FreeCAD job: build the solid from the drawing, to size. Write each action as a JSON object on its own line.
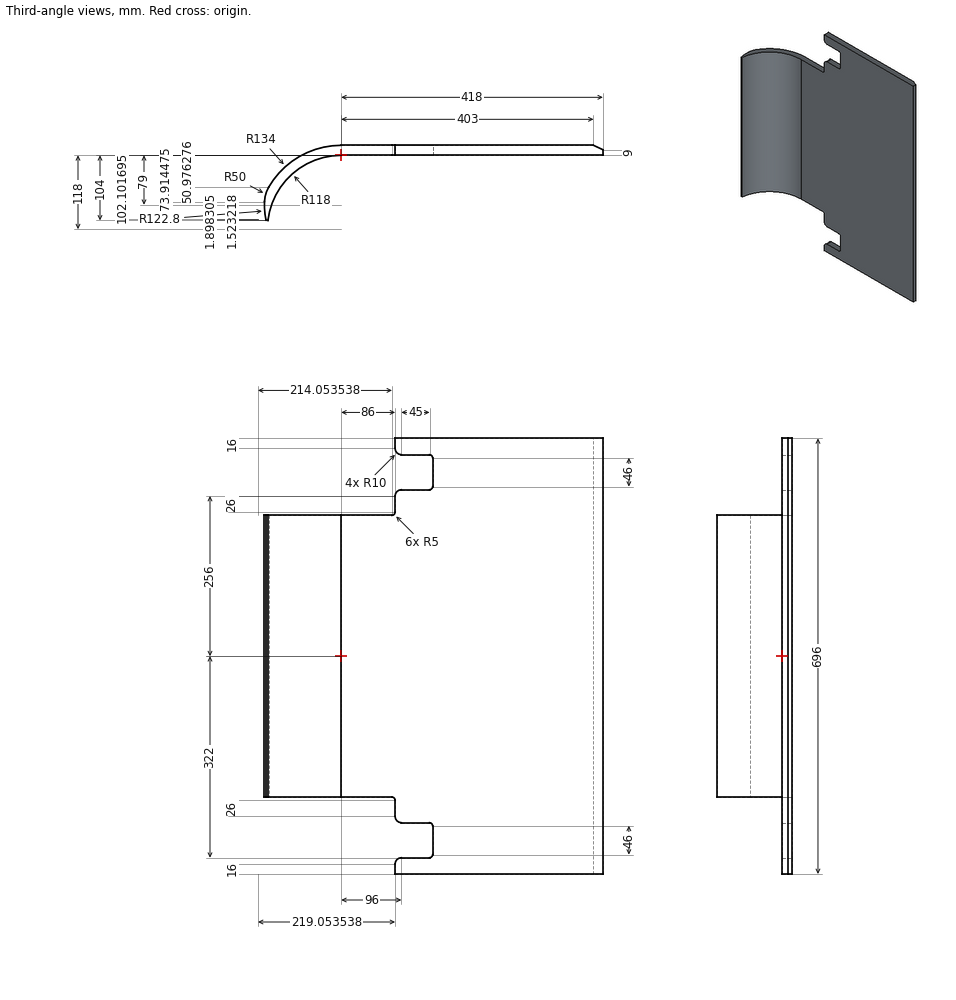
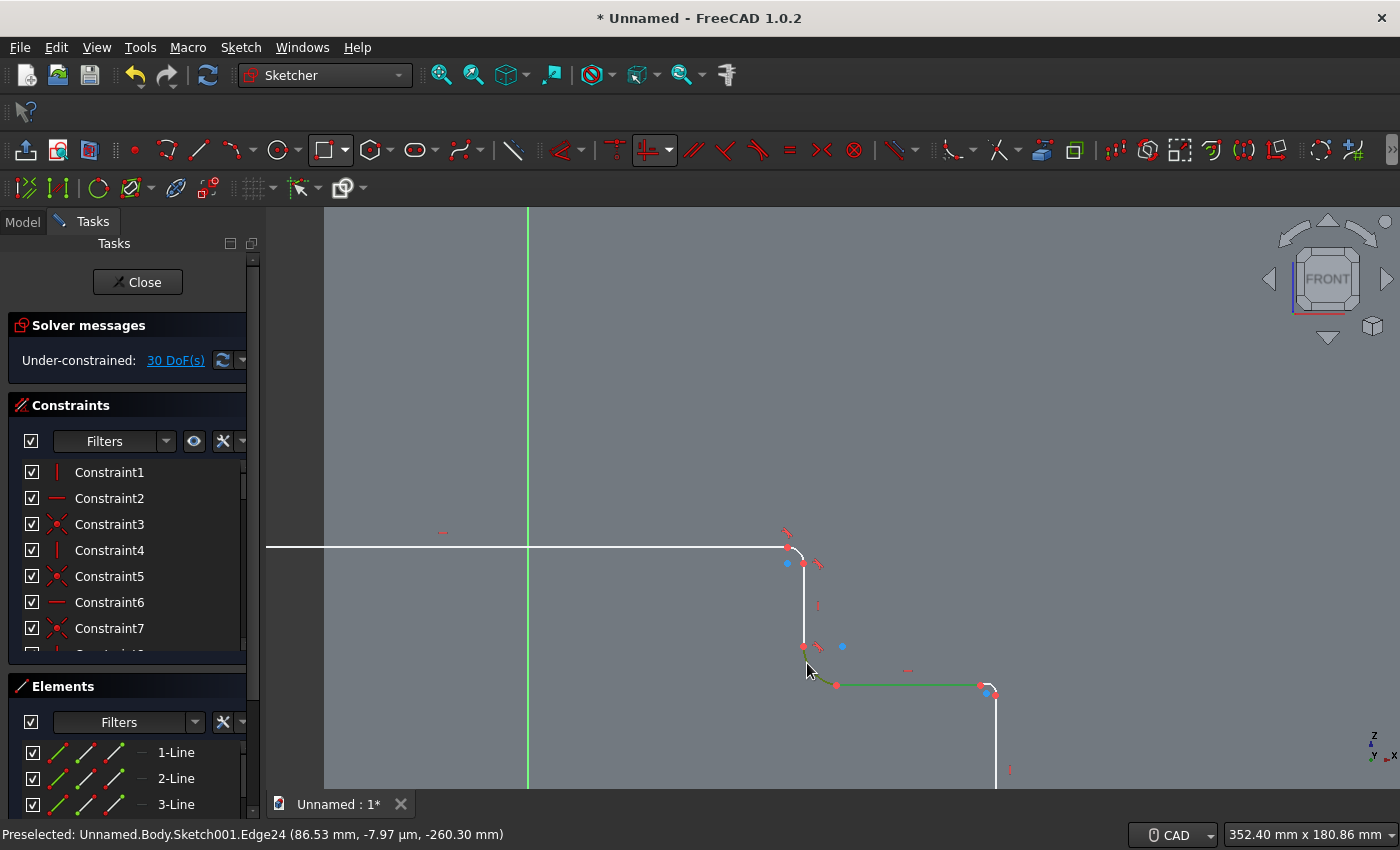
{"action": "left_click", "coordinate": [758, 150]}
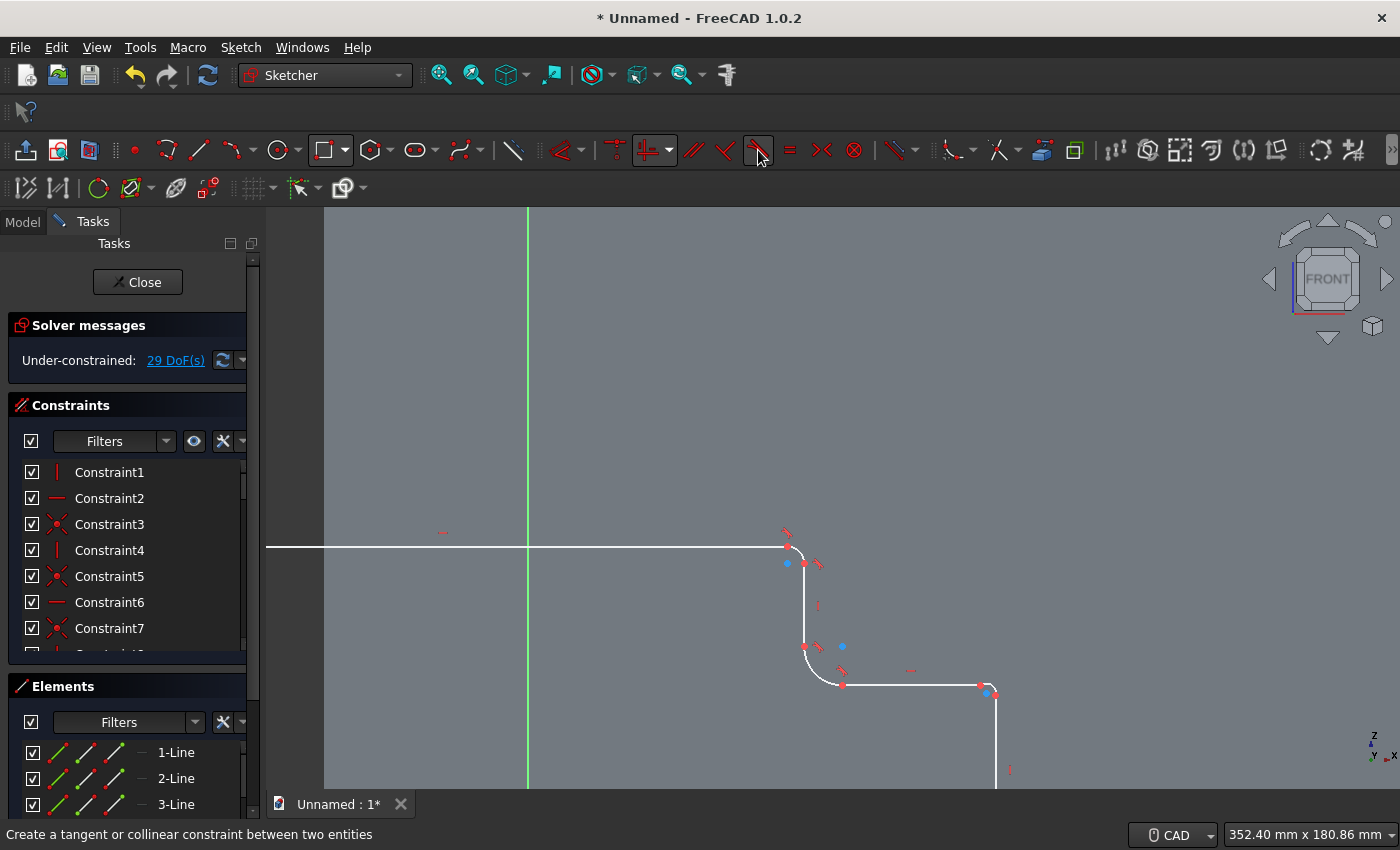
{"action": "scroll", "coordinate": [807, 632], "scroll_direction": "down", "scroll_amount": 9}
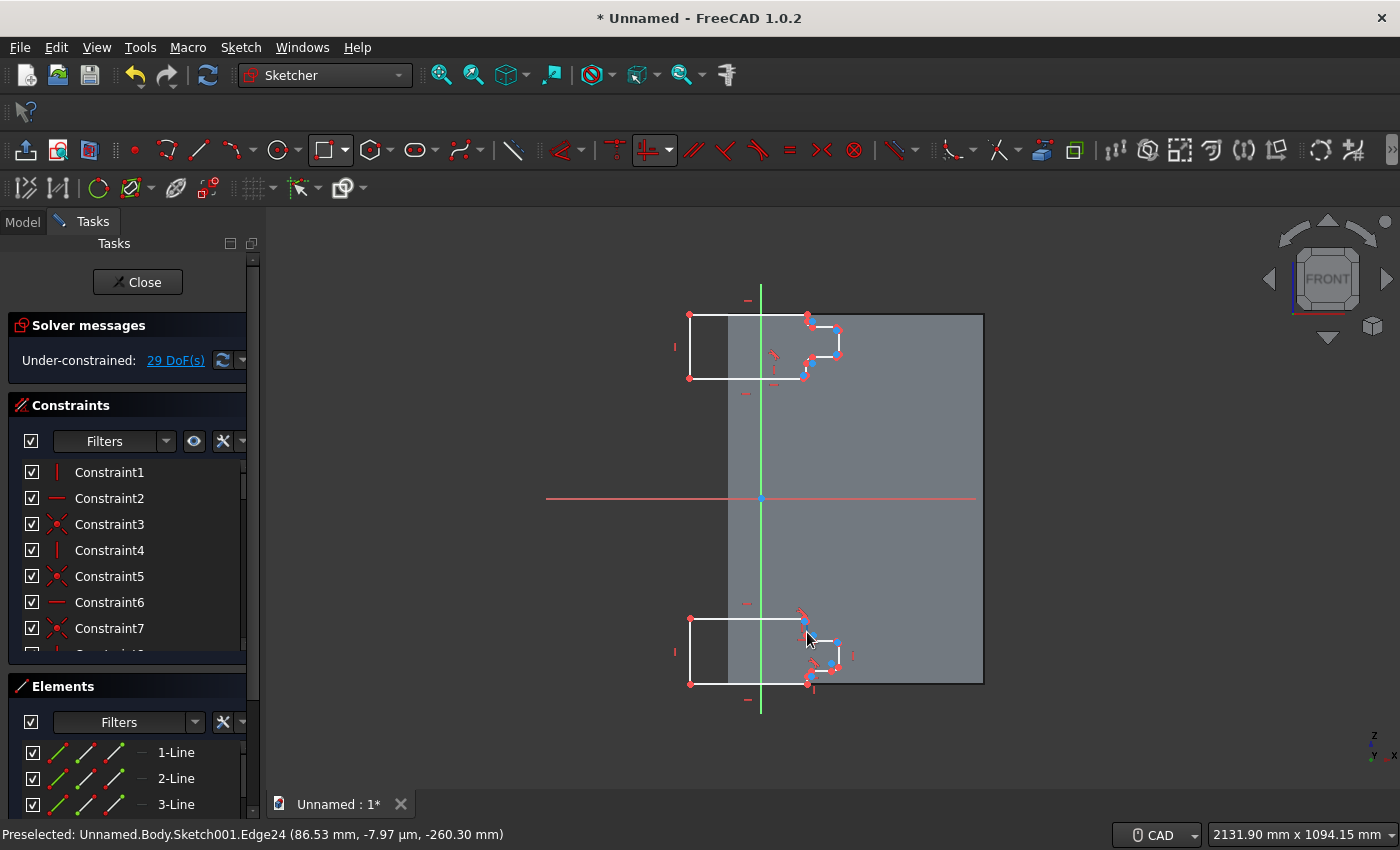
{"action": "scroll", "coordinate": [820, 641], "scroll_direction": "up", "scroll_amount": 4}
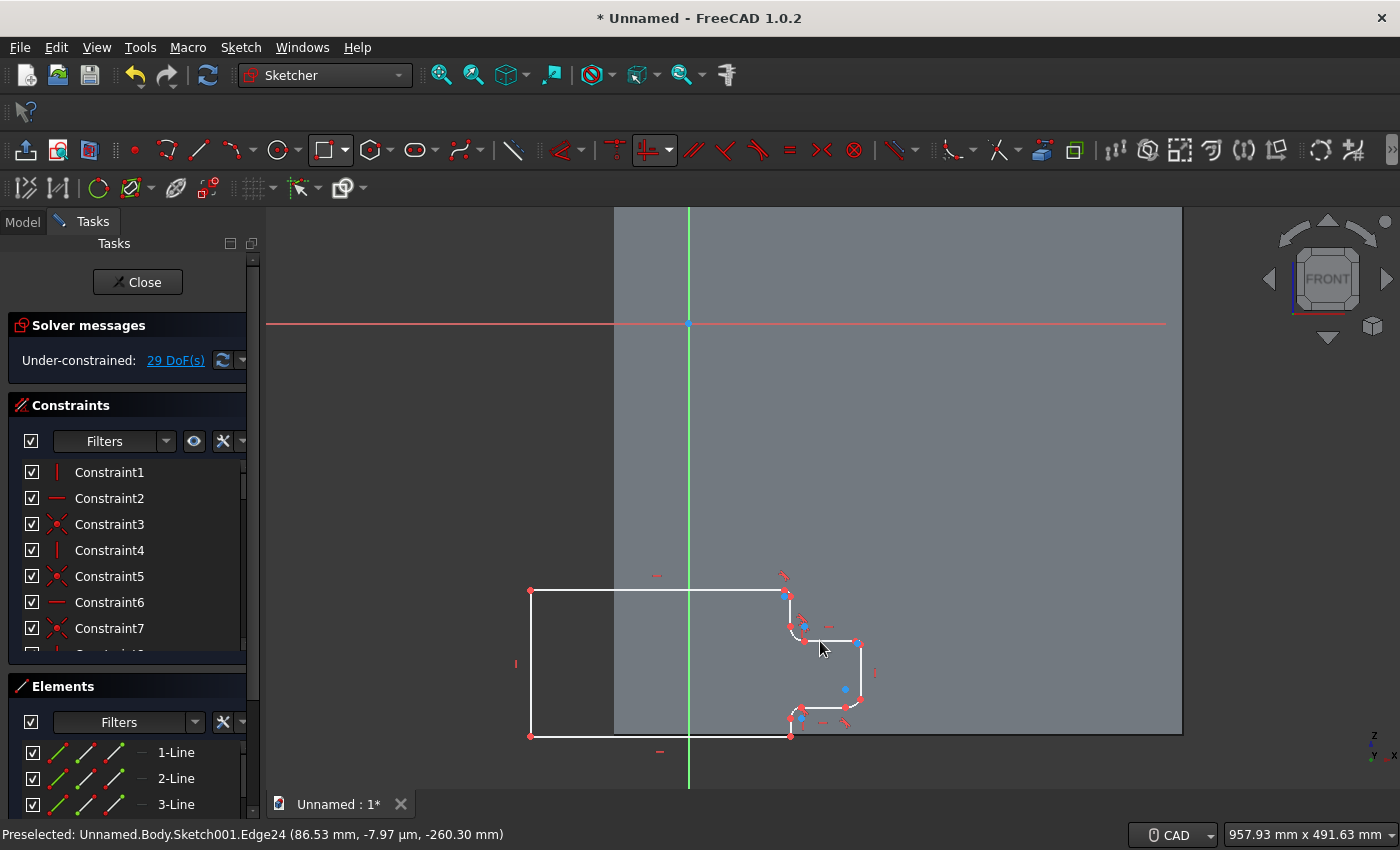
{"action": "left_click", "coordinate": [820, 641]}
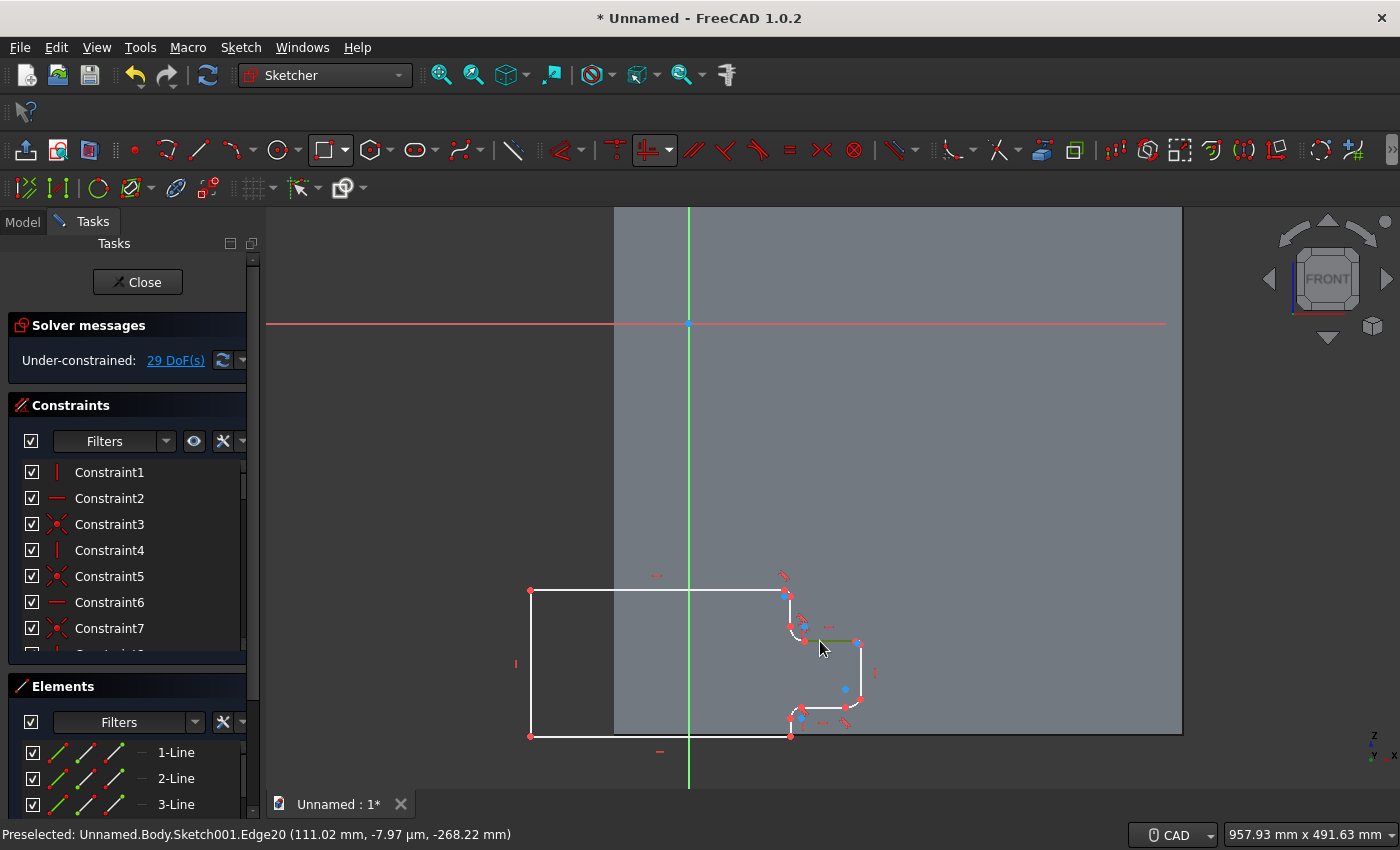
{"action": "scroll", "coordinate": [859, 641], "scroll_direction": "up", "scroll_amount": 7}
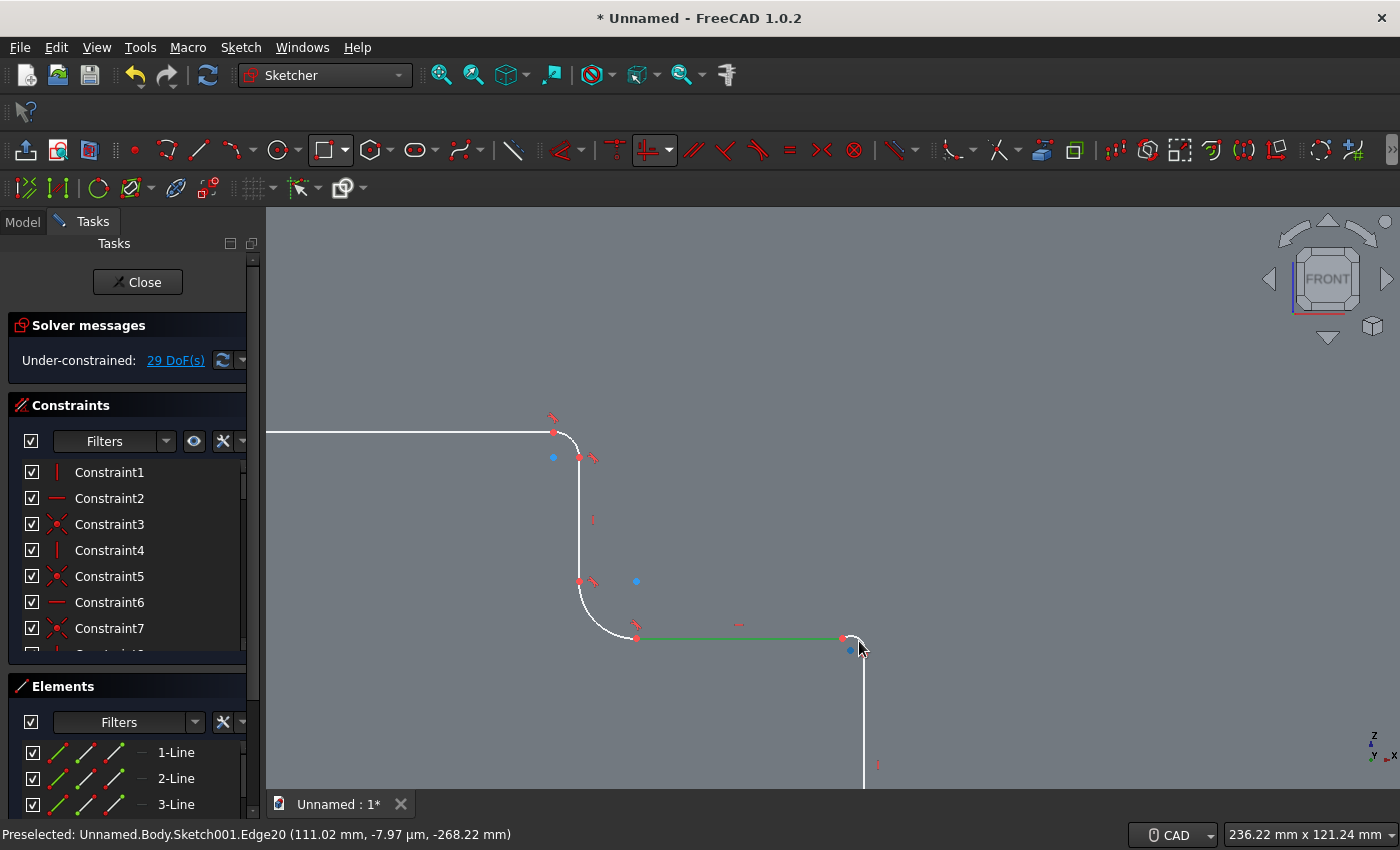
{"action": "left_click", "coordinate": [859, 639]}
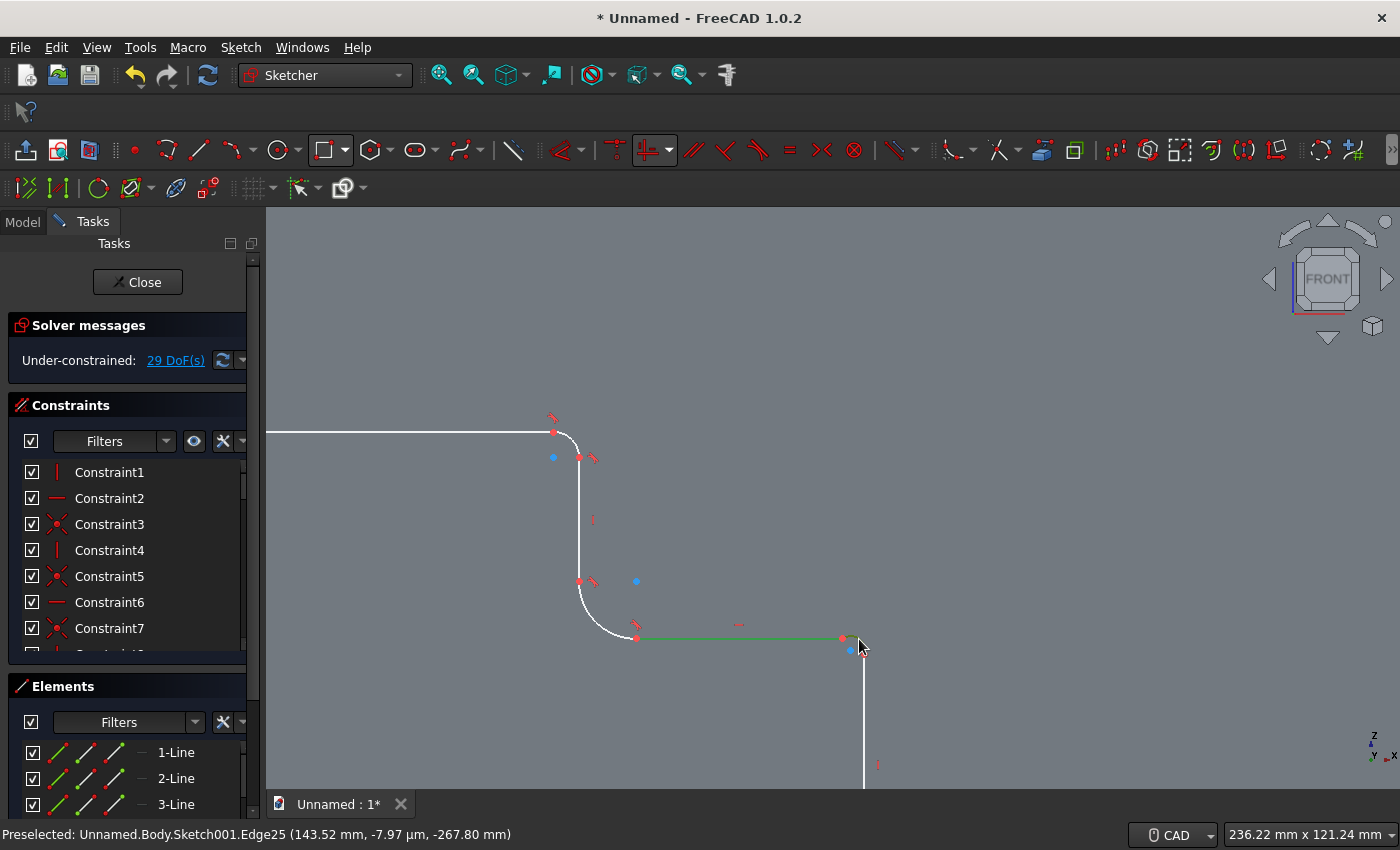
{"action": "left_click", "coordinate": [758, 150]}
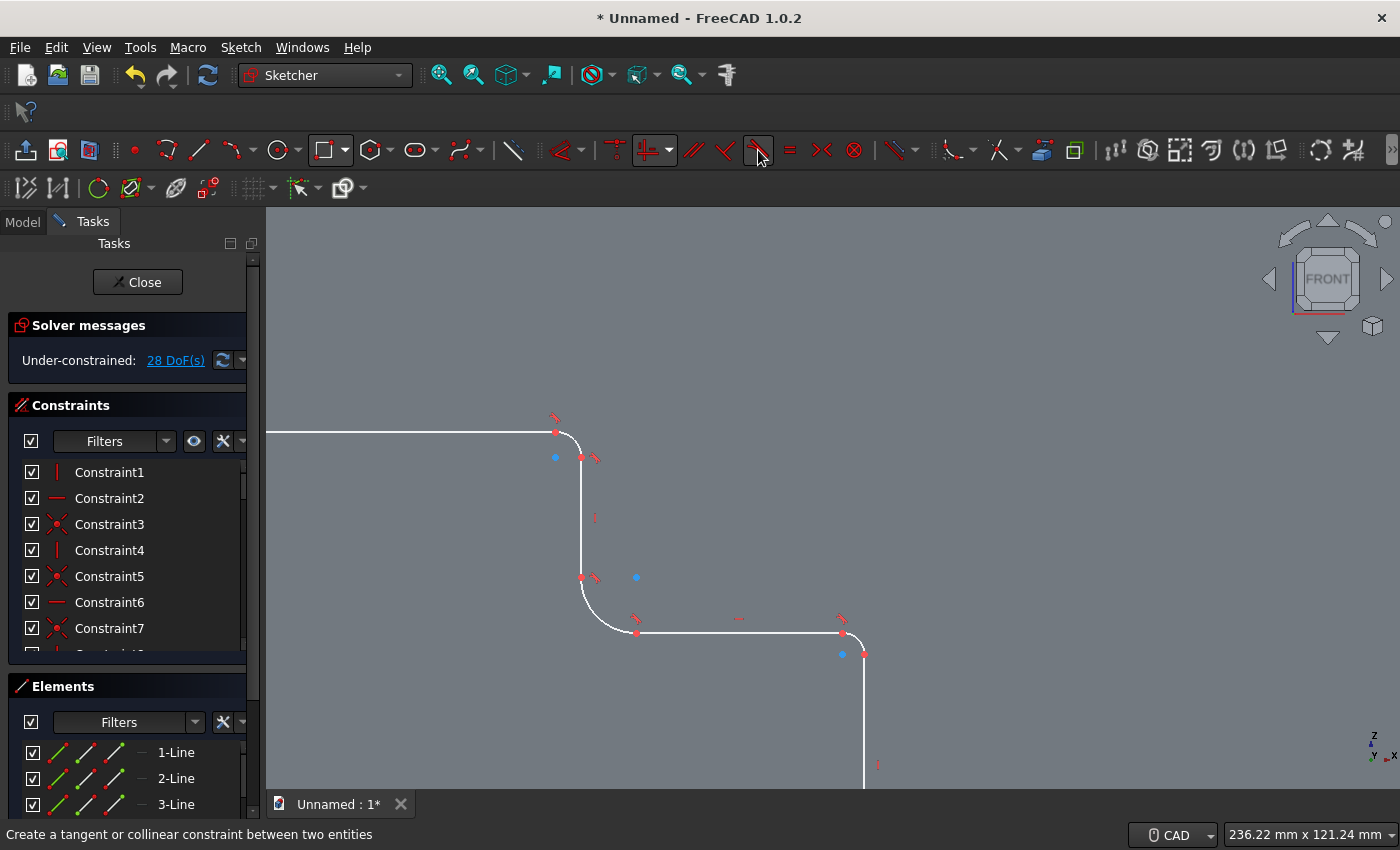
{"action": "scroll", "coordinate": [835, 641], "scroll_direction": "down", "scroll_amount": 11}